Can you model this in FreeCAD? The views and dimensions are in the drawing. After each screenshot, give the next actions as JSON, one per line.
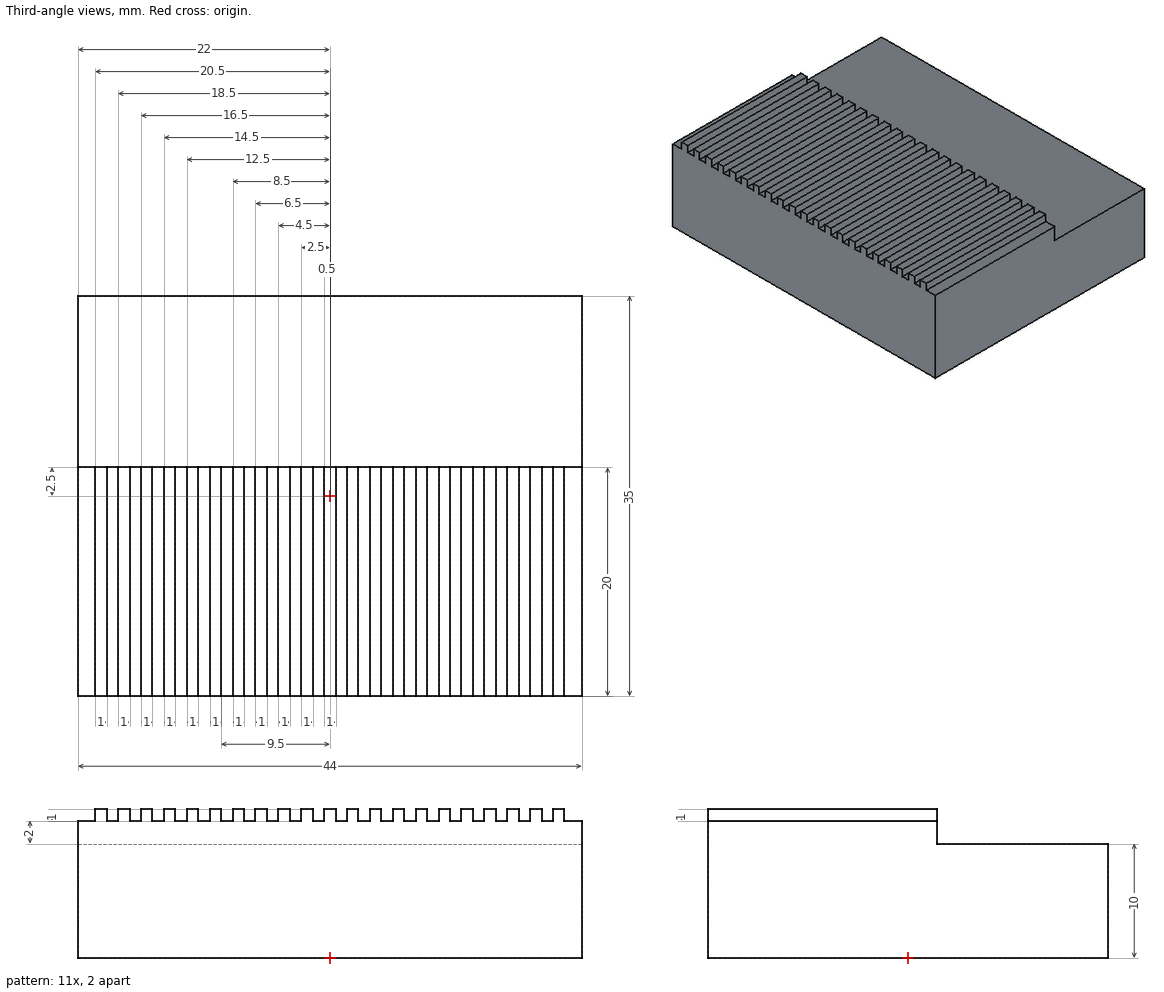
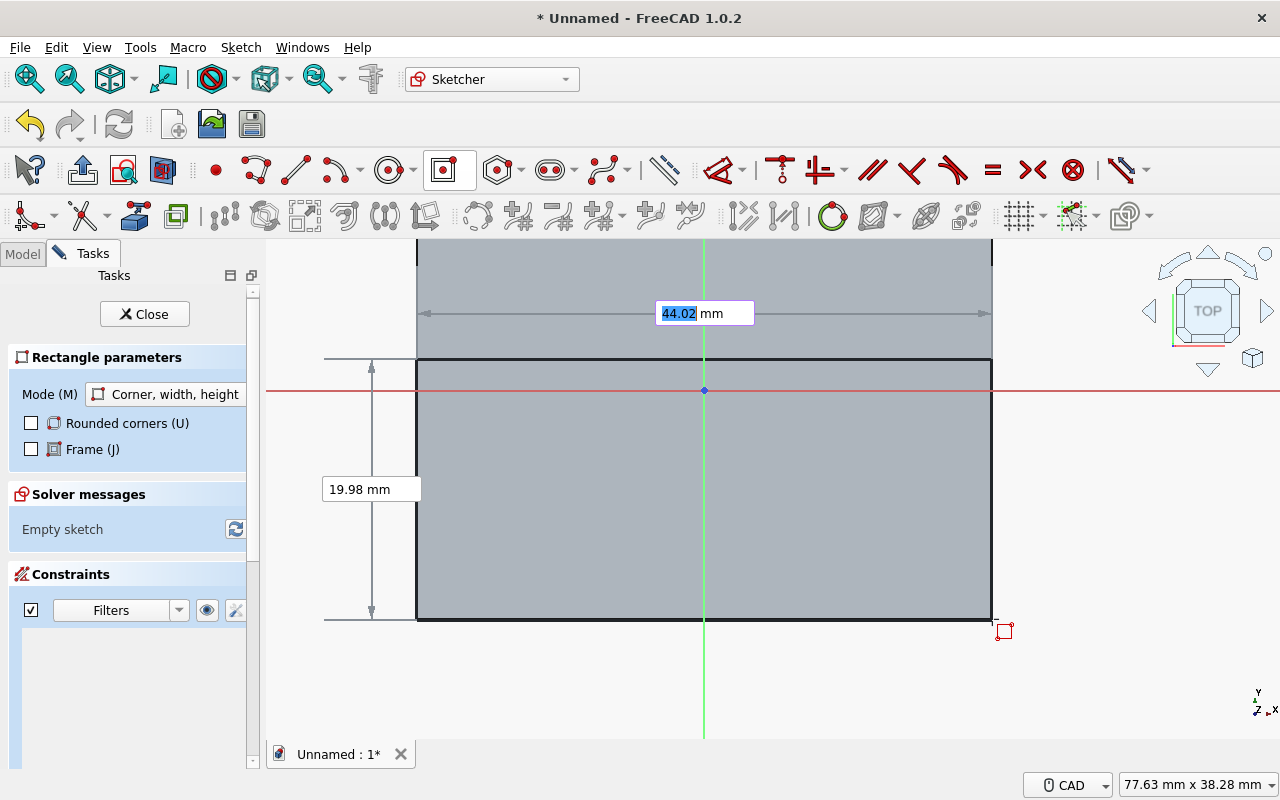
{"action": "type", "text": "44"}
{"action": "key", "text": "Tab"}
{"action": "type", "text": "20"}
{"action": "key", "text": "Return"}
{"action": "key", "text": "Escape"}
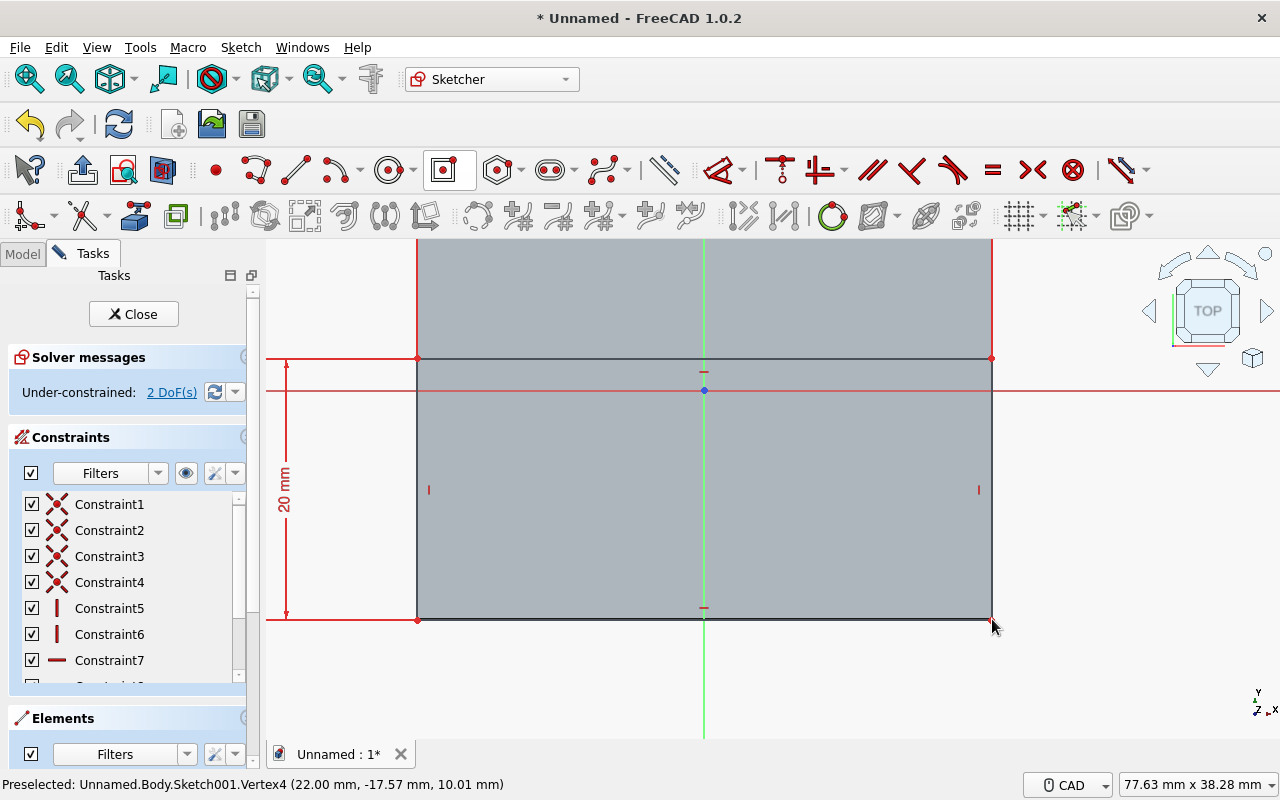
{"action": "left_click", "coordinate": [417, 359]}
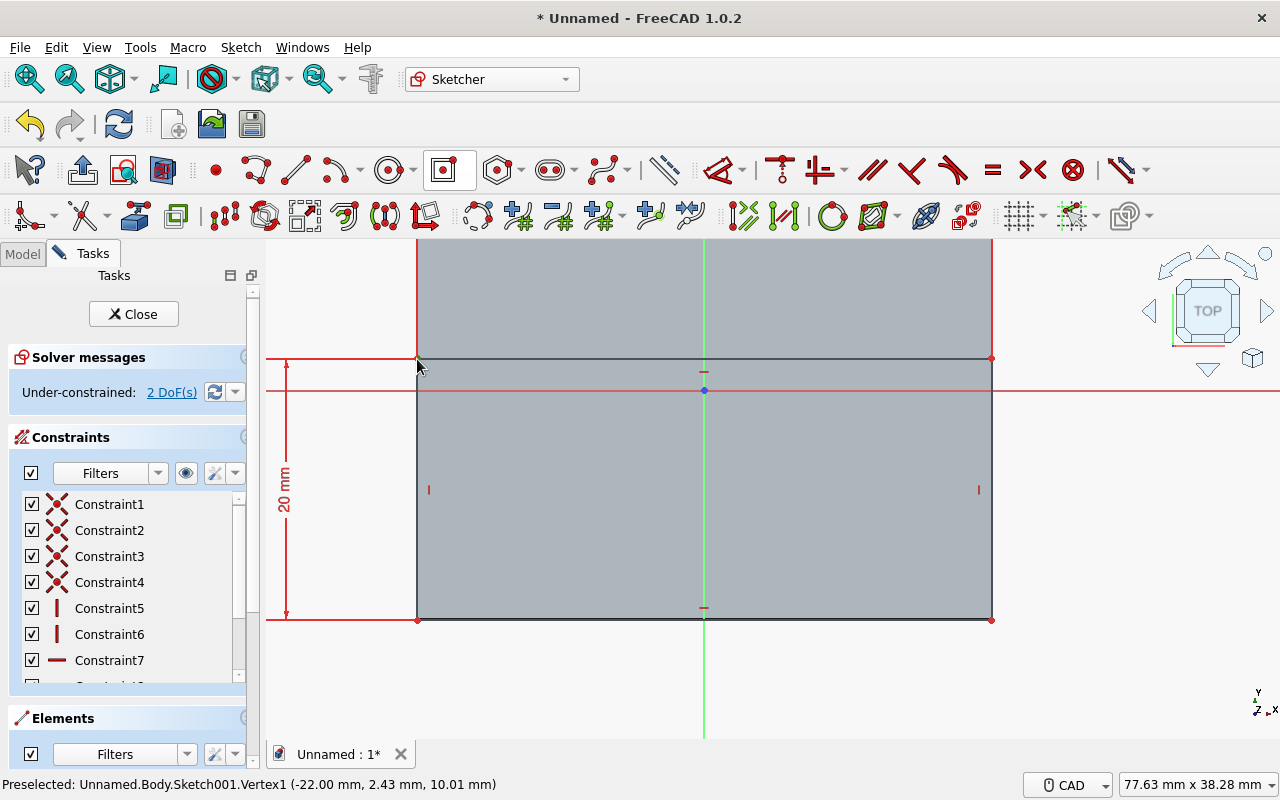
{"action": "key", "text": "l"}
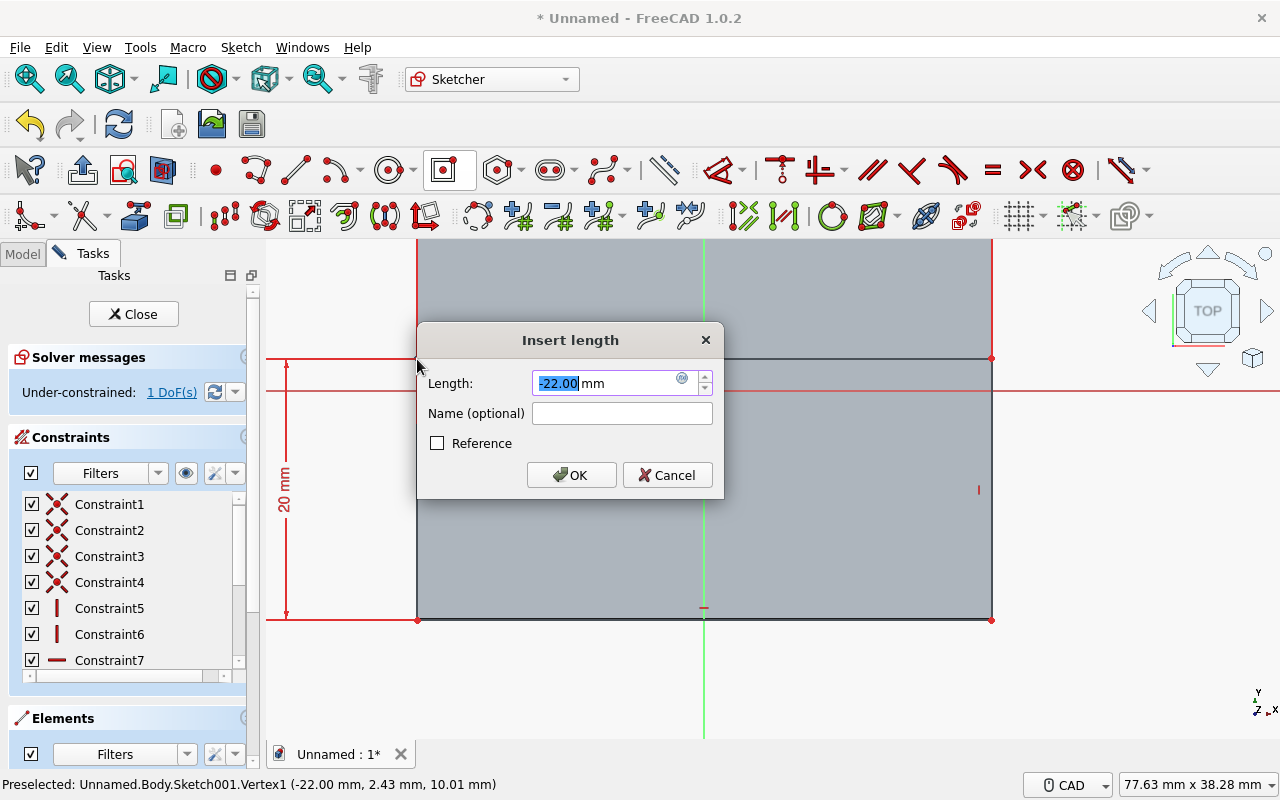
{"action": "type", "text": "-22"}
{"action": "key", "text": "Return"}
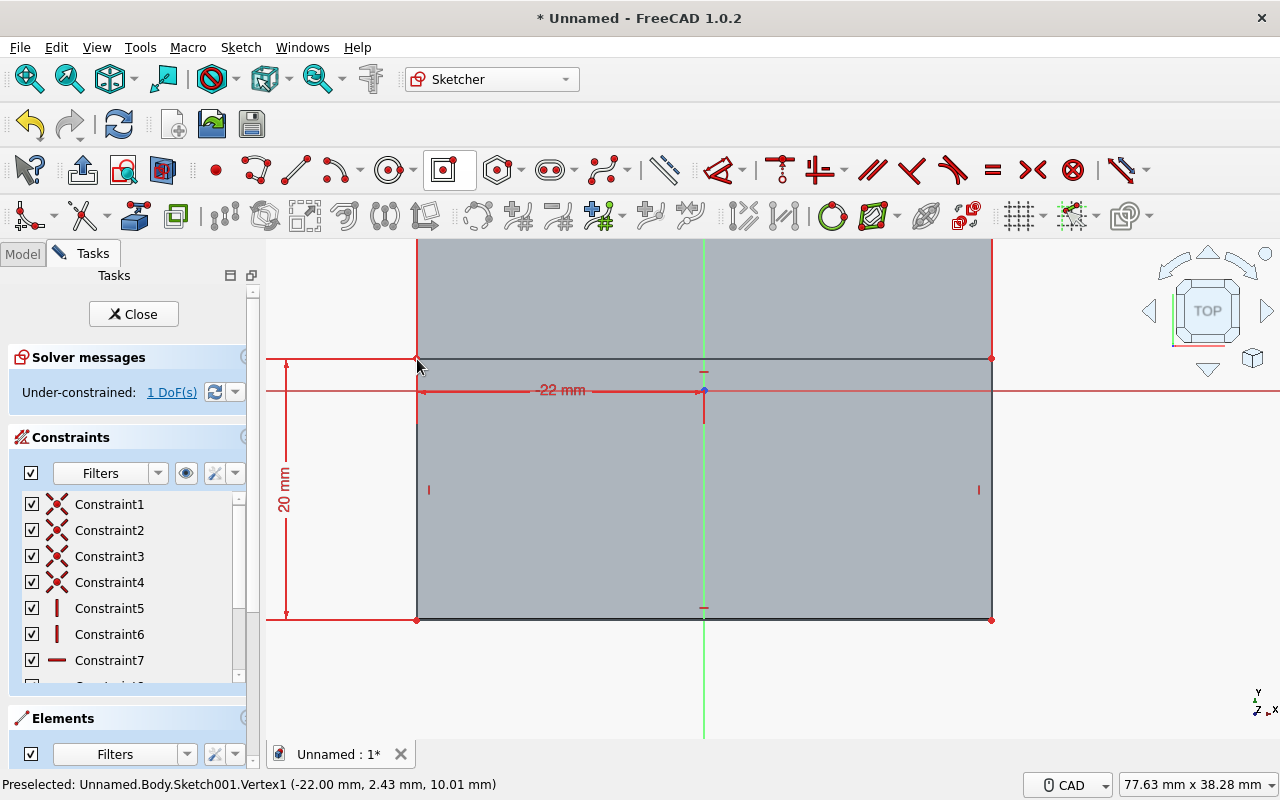
{"action": "left_click", "coordinate": [417, 359]}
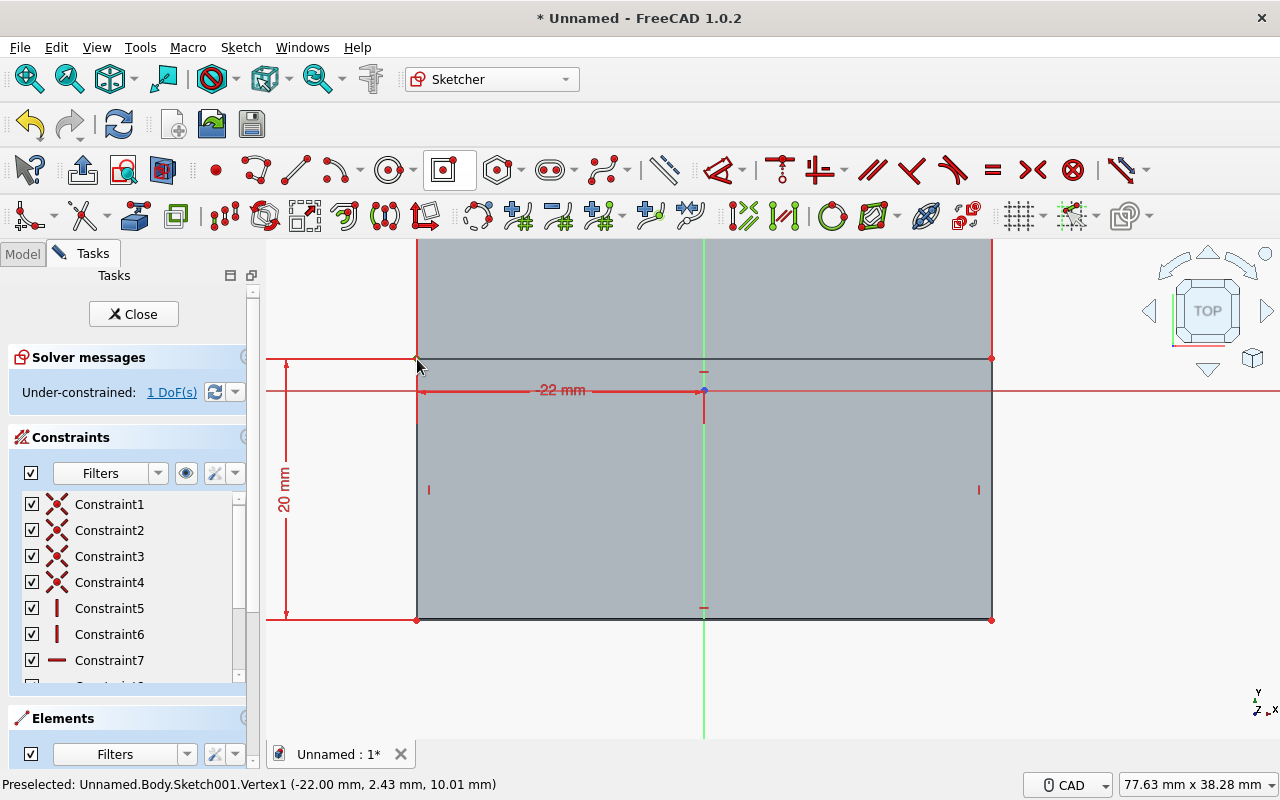
{"action": "key", "text": "i"}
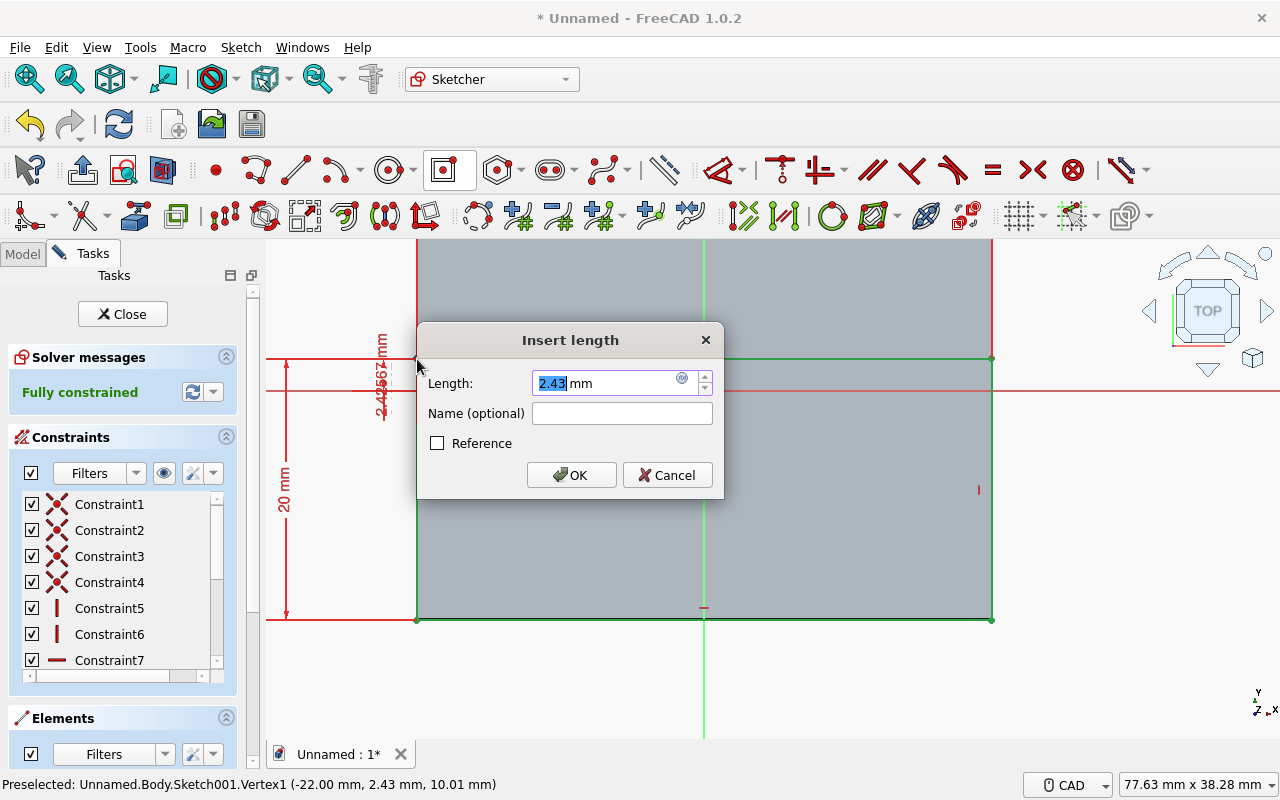
{"action": "type", "text": "2.5"}
{"action": "key", "text": "Return"}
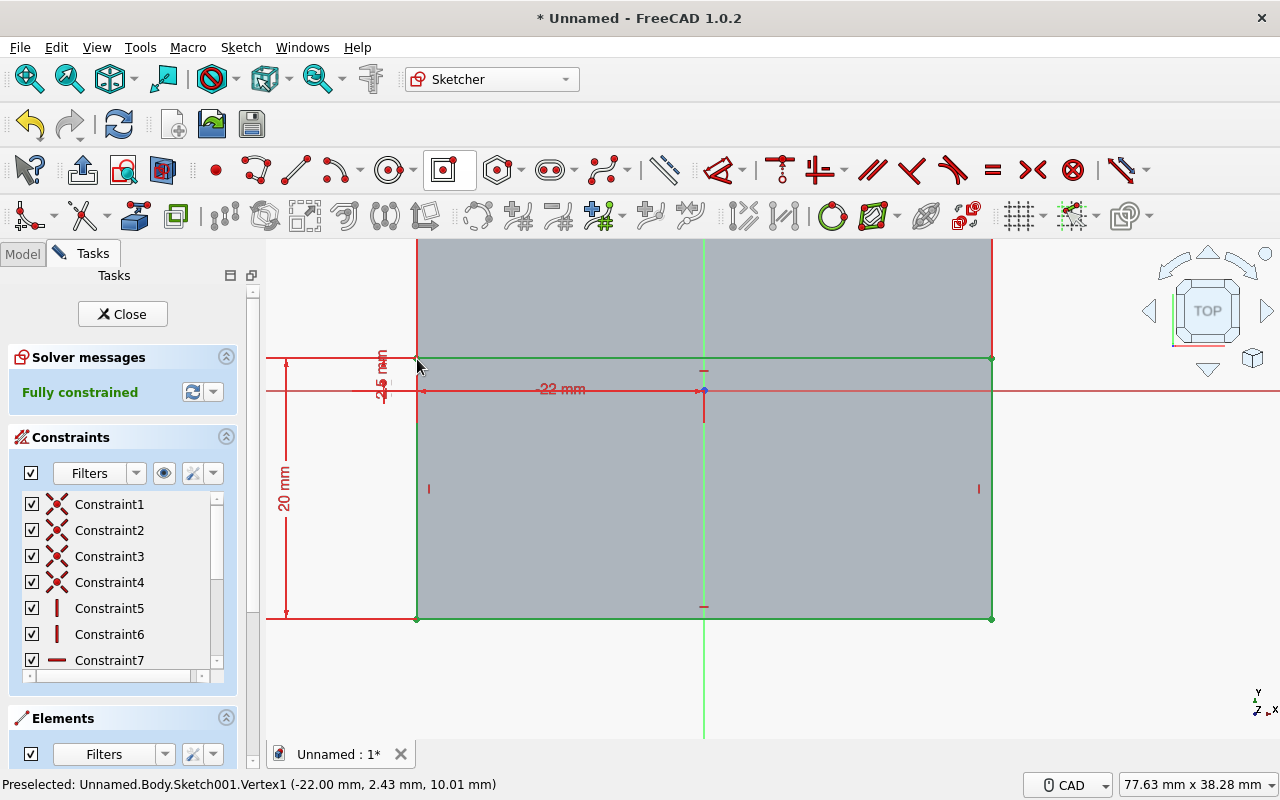
{"action": "left_click", "coordinate": [123, 314]}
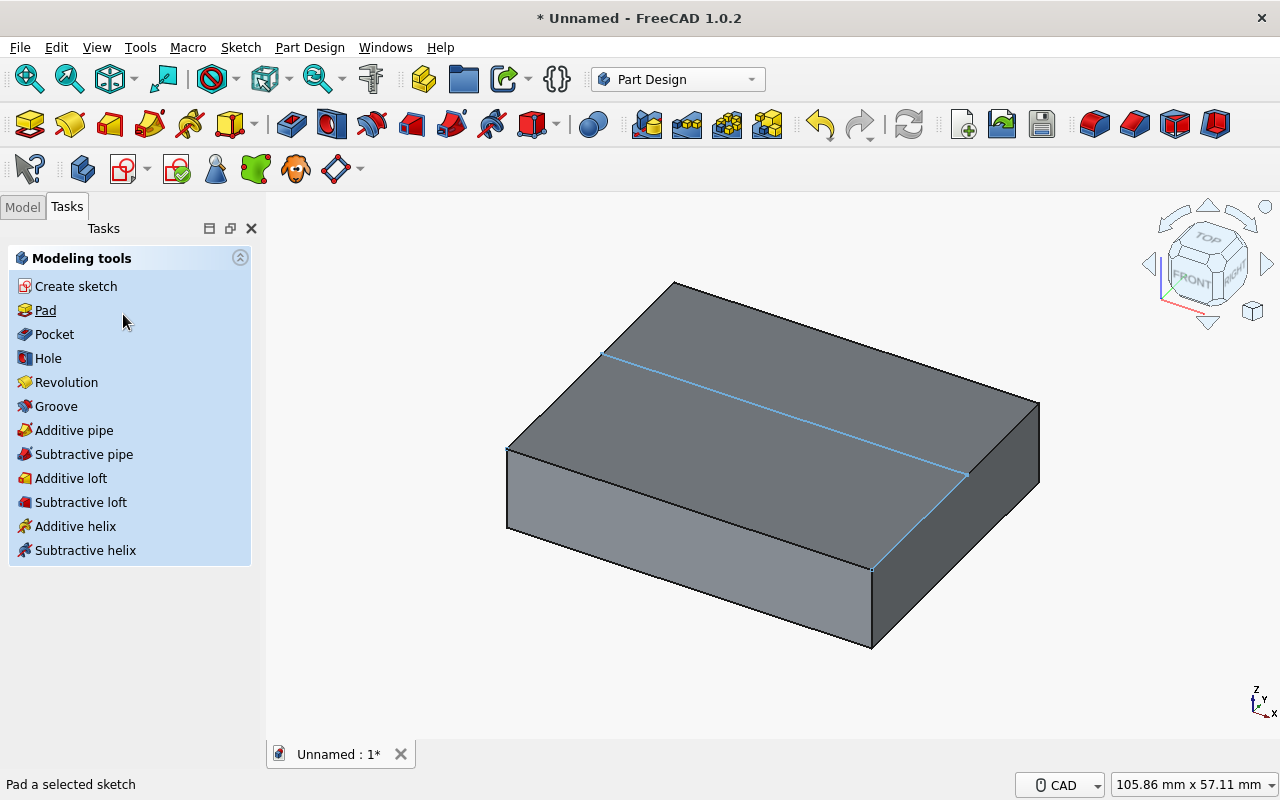
{"action": "left_click", "coordinate": [30, 124]}